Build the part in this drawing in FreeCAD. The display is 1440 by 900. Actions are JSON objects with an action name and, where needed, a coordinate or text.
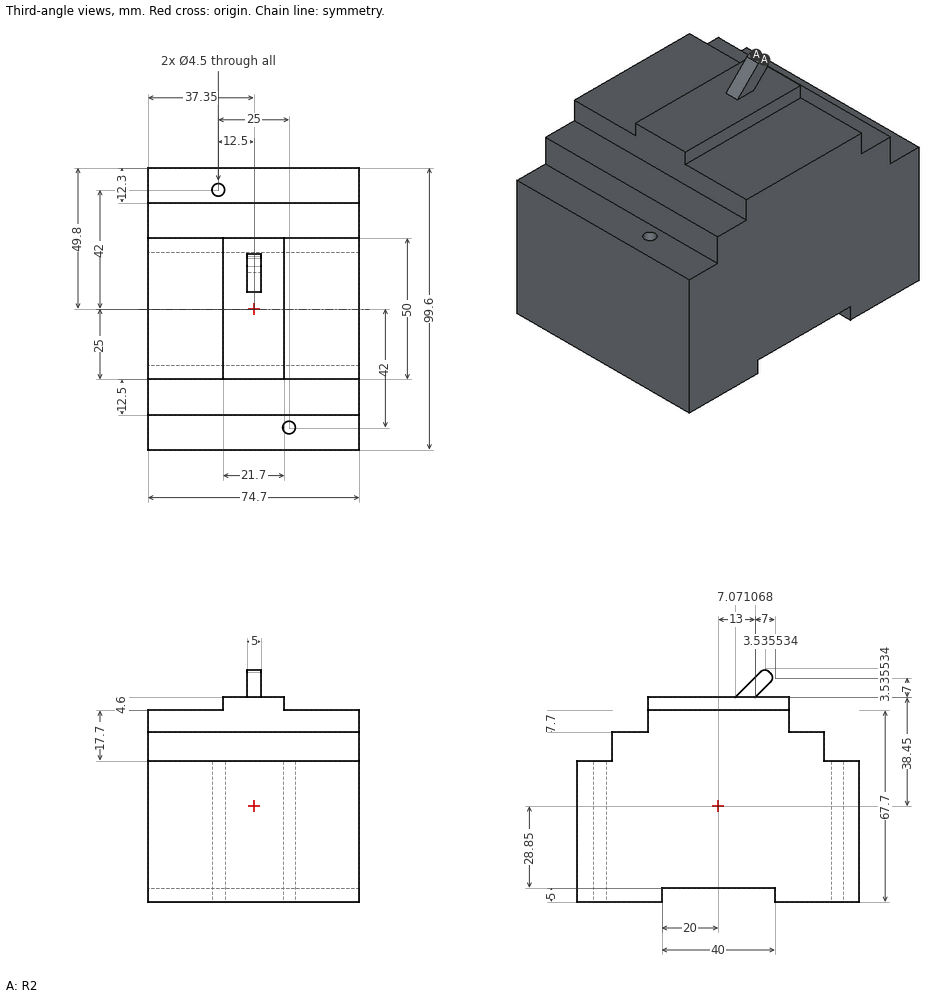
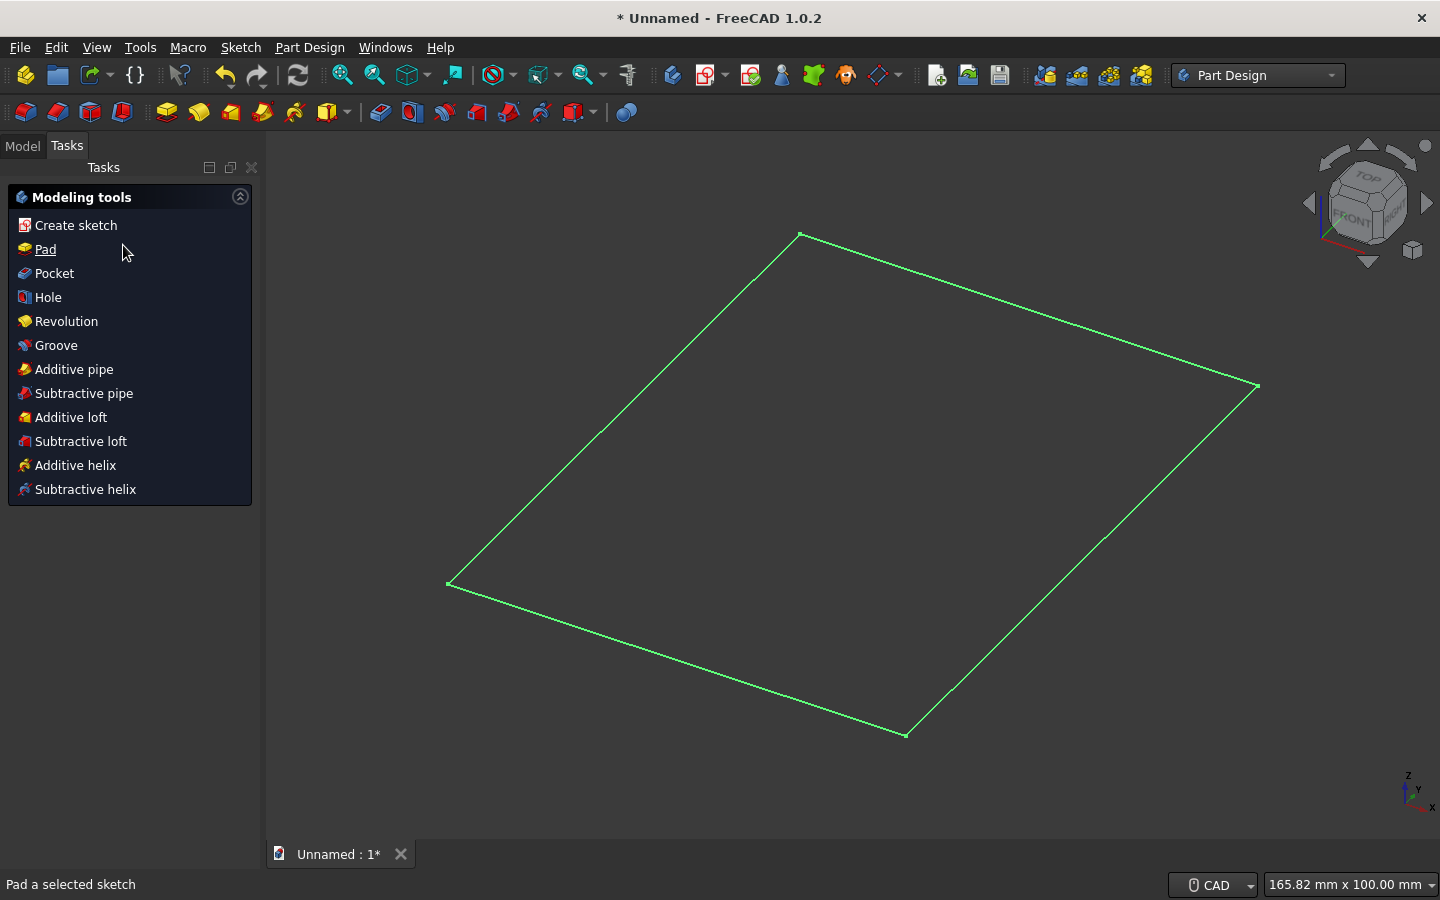
{"action": "left_click", "coordinate": [168, 112]}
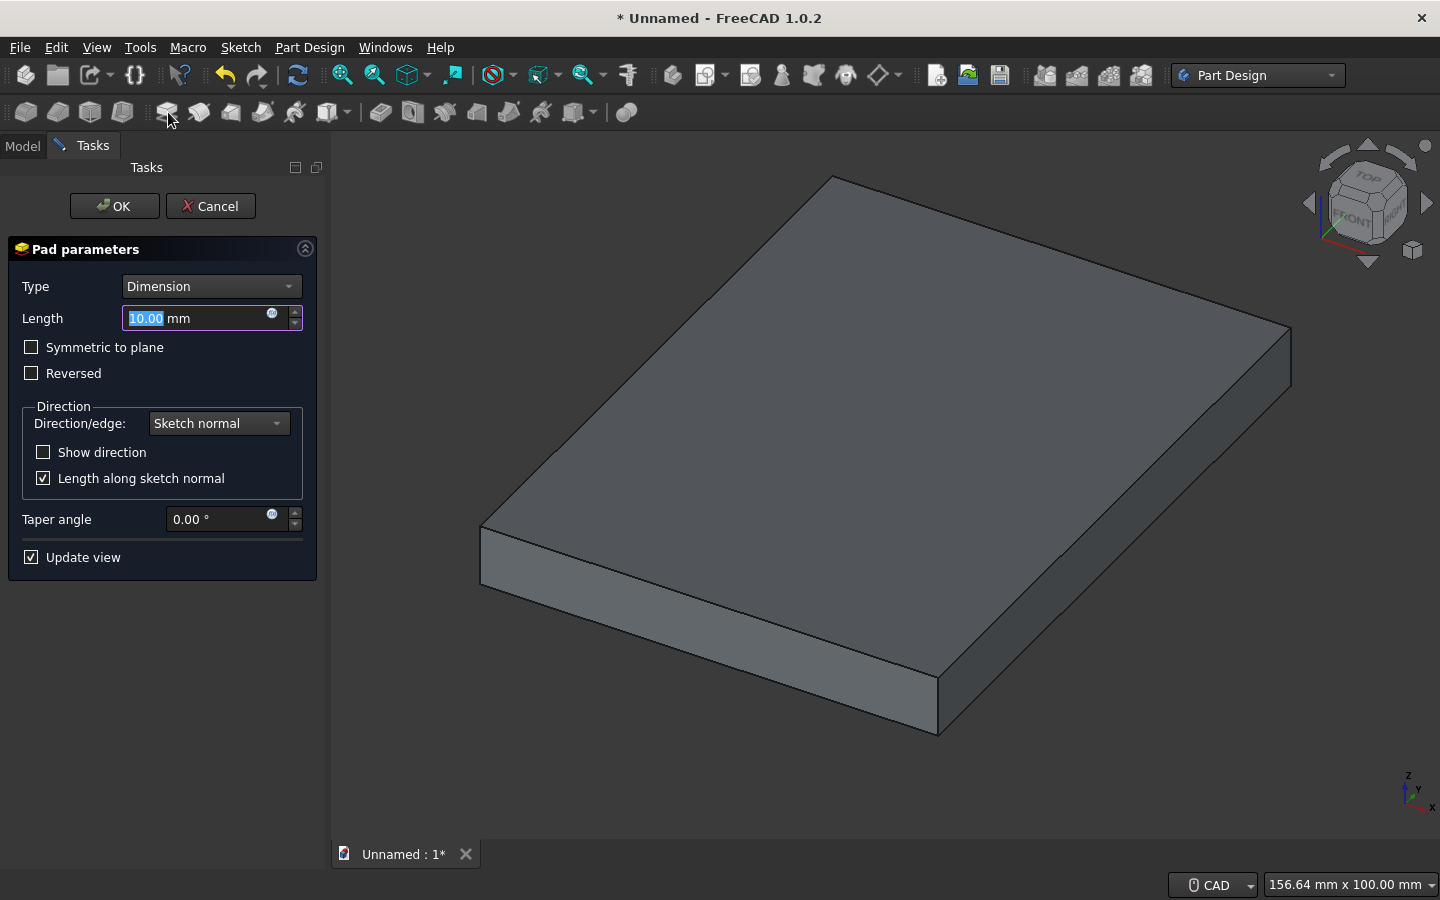
{"action": "type", "text": "67.7"}
{"action": "key", "text": "Tab"}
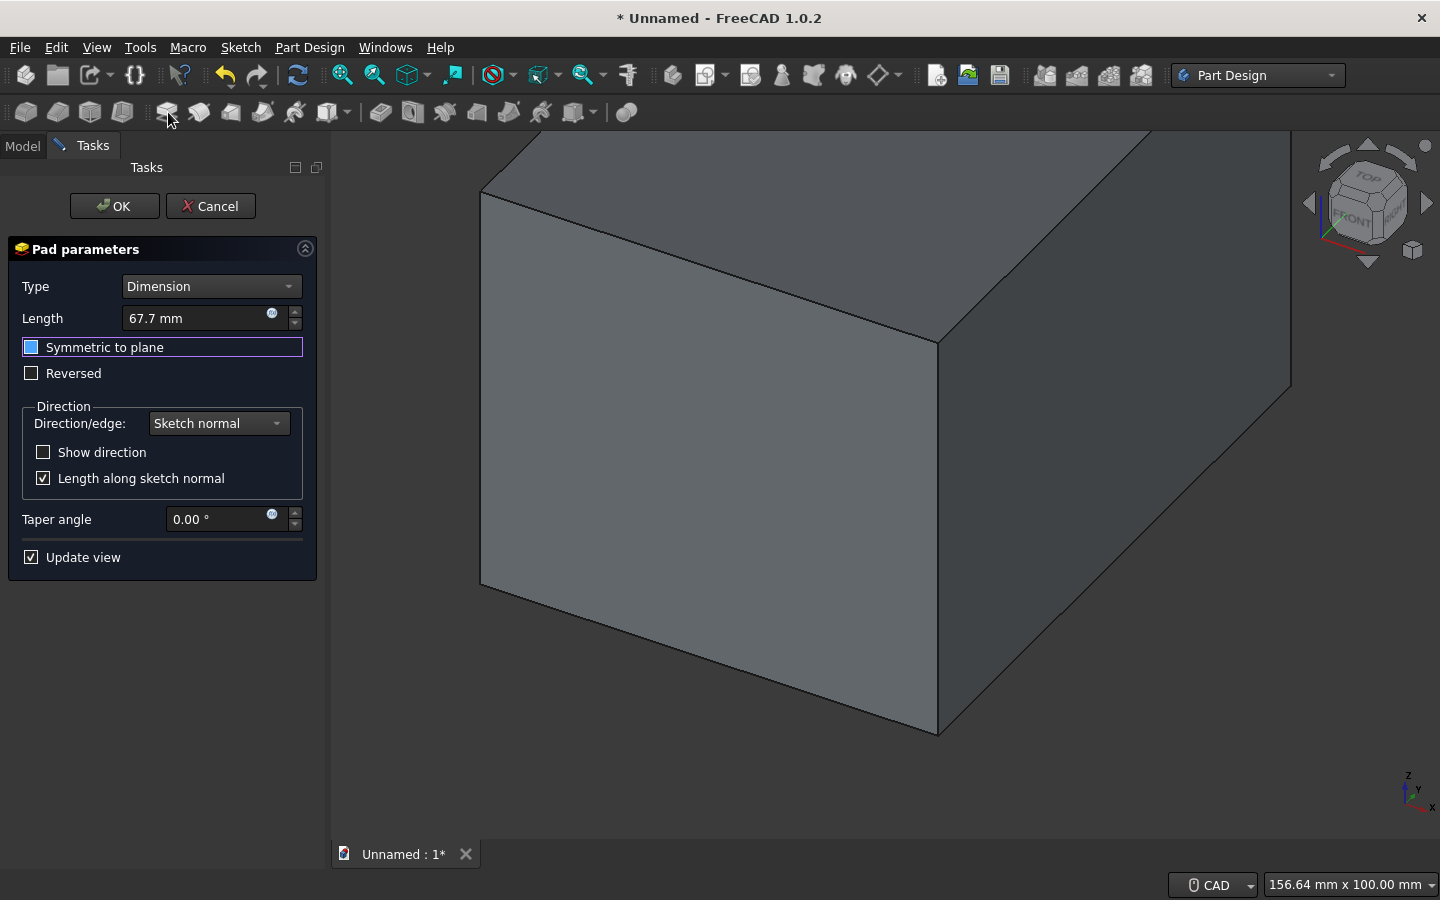
{"action": "left_click", "coordinate": [30, 347]}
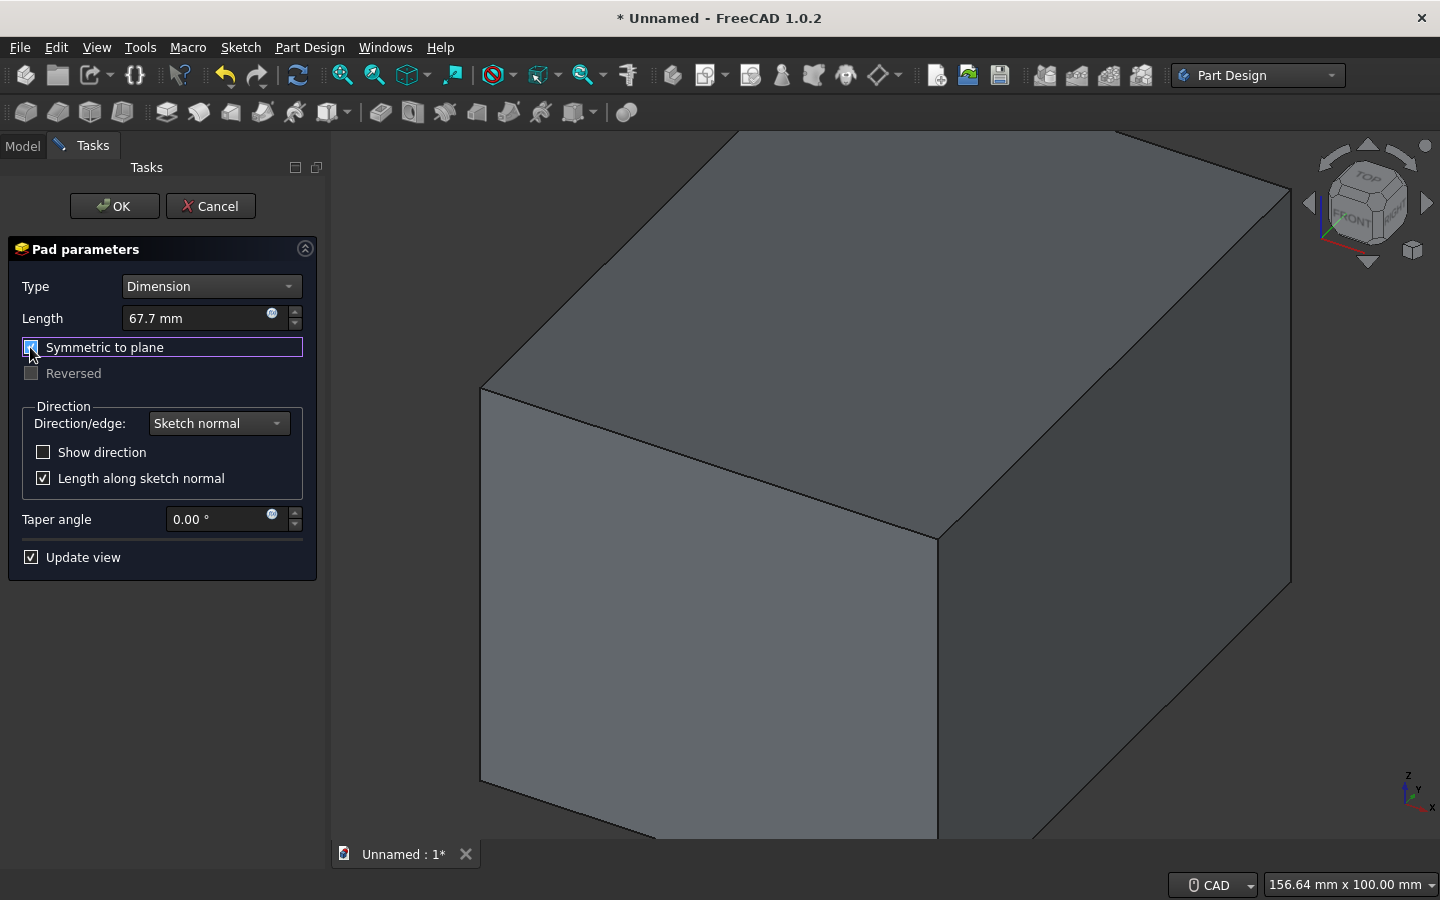
{"action": "left_click", "coordinate": [115, 206]}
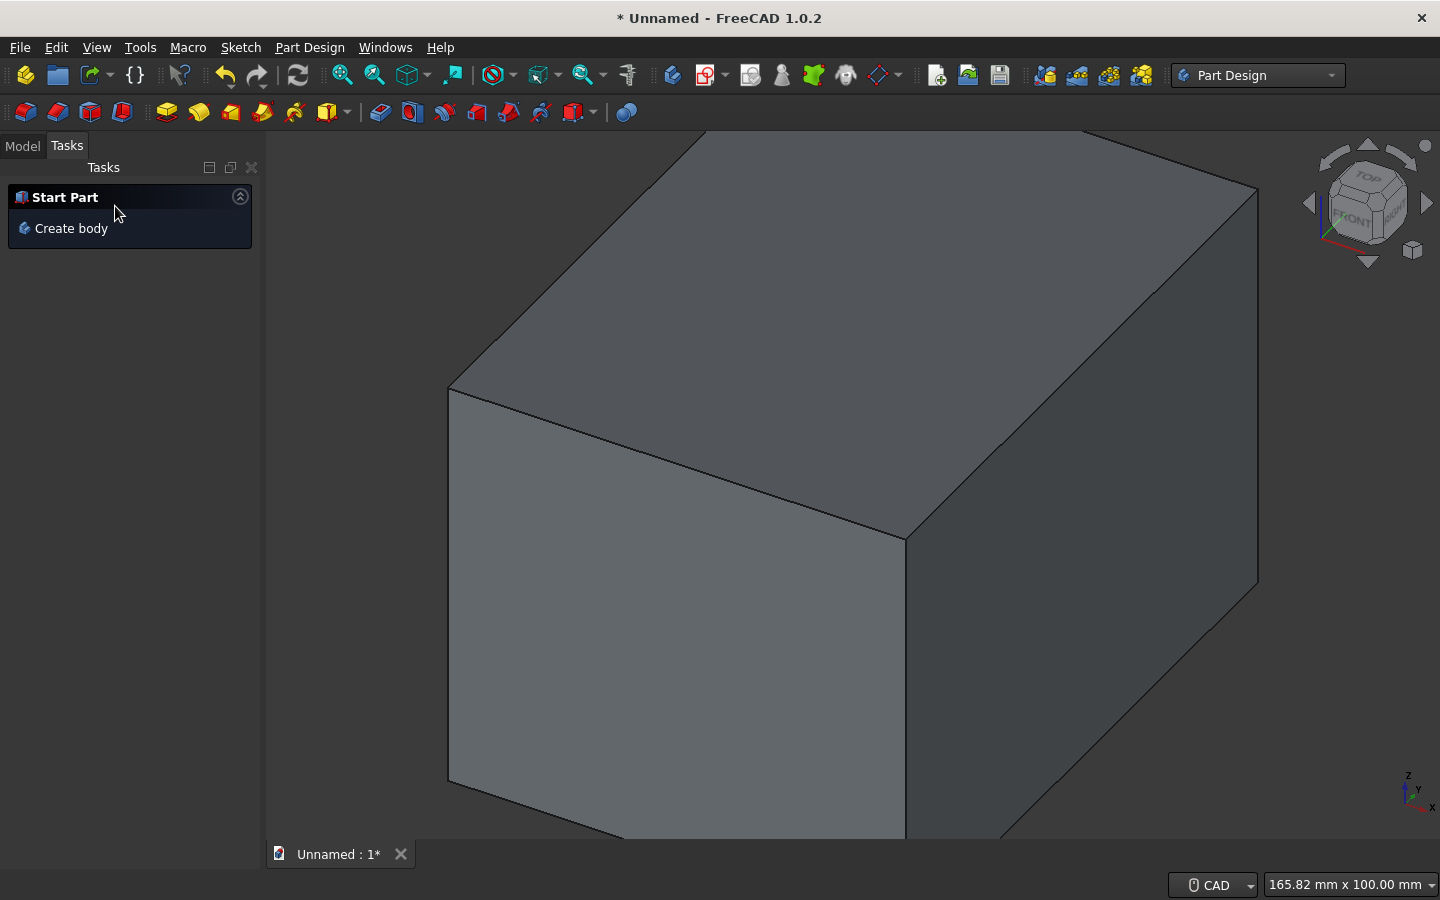
{"action": "left_click", "coordinate": [344, 76]}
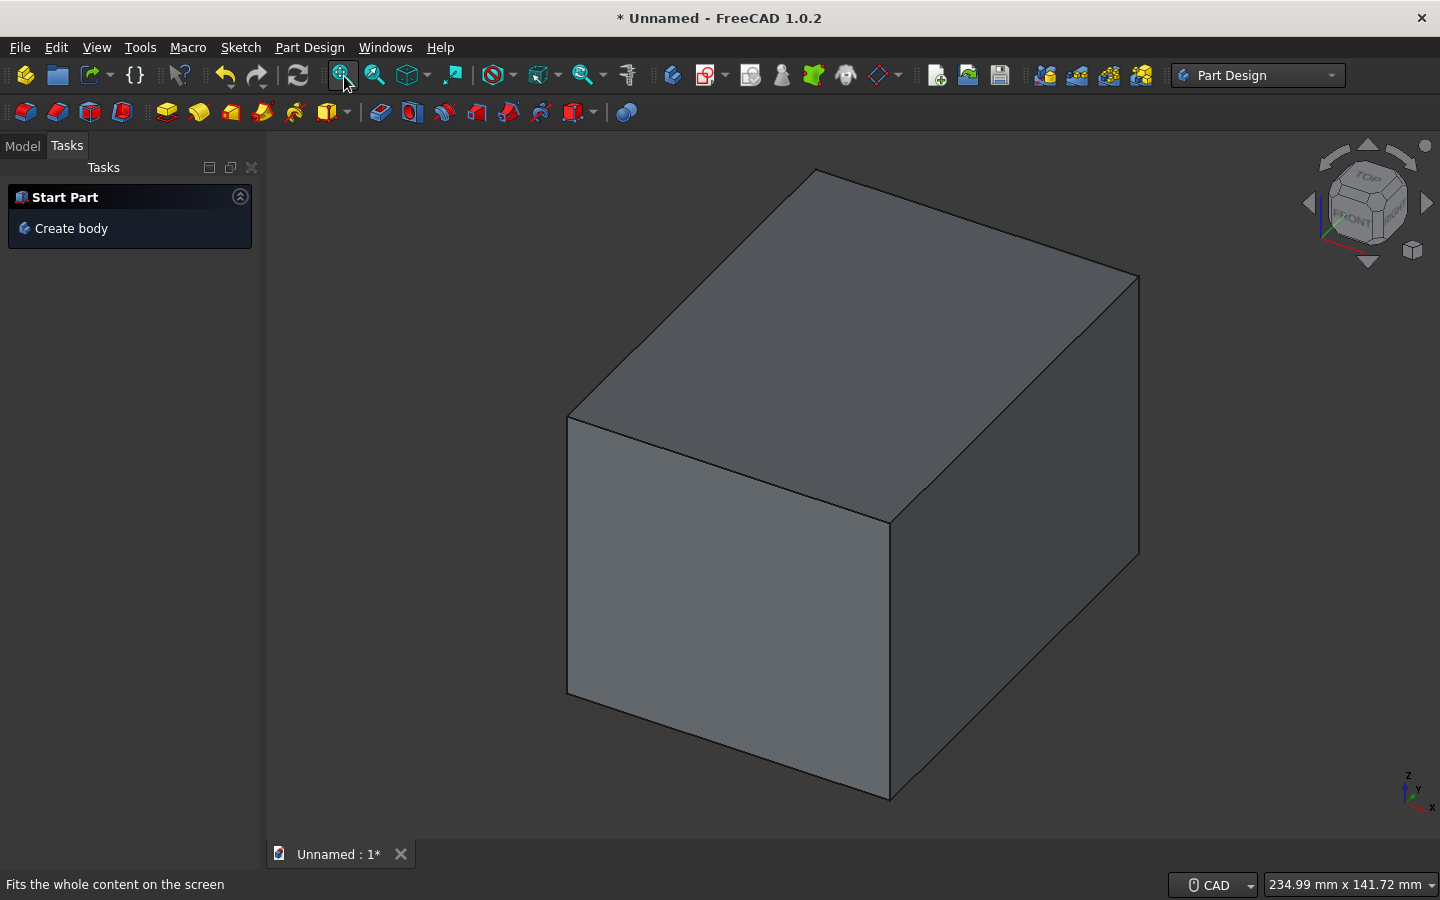
{"action": "left_click", "coordinate": [853, 345]}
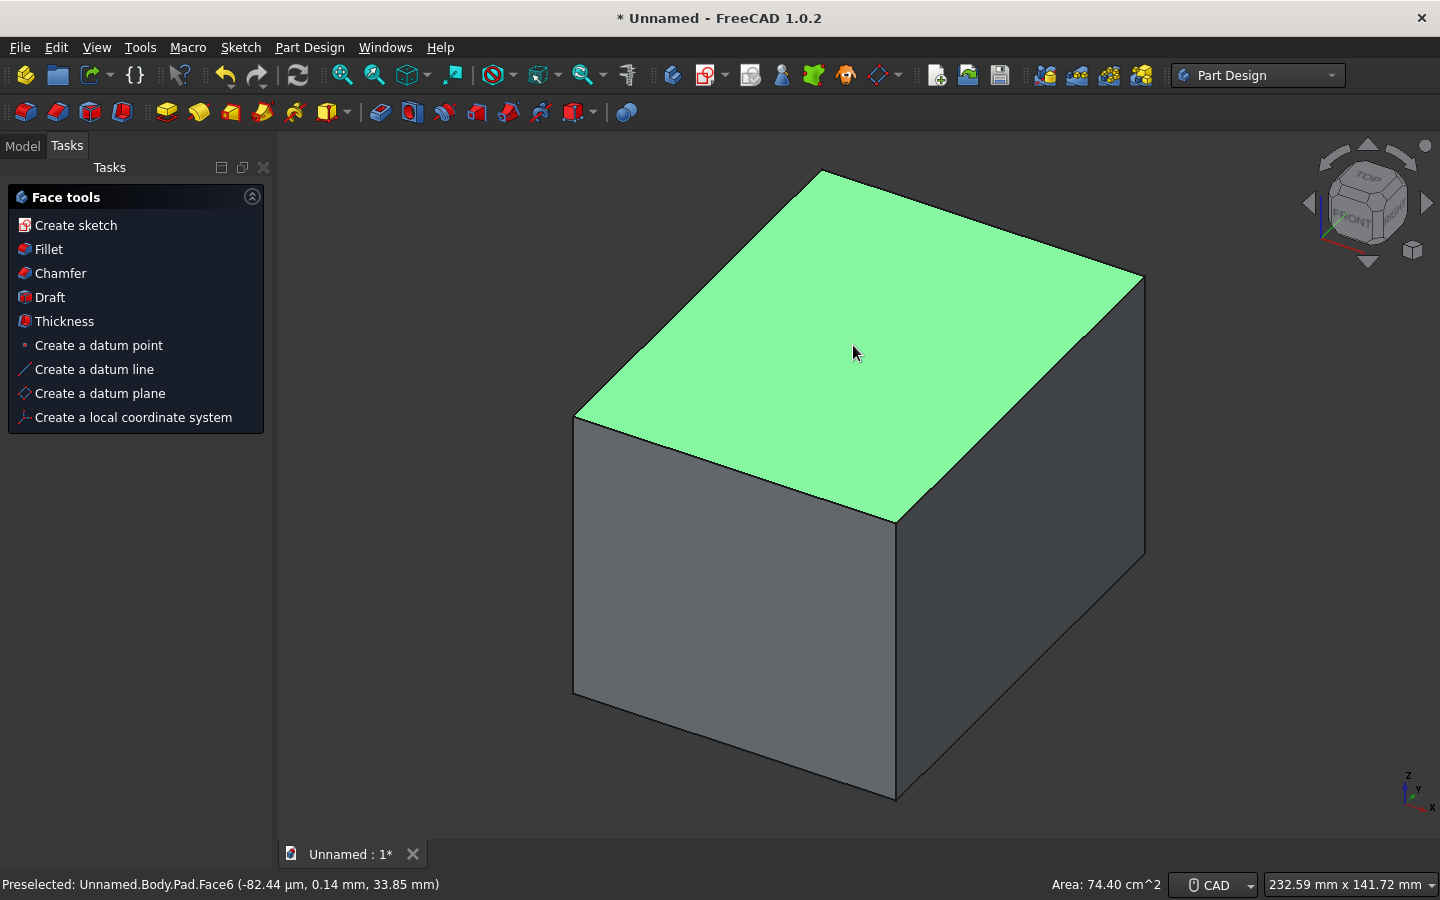
{"action": "left_click", "coordinate": [706, 76]}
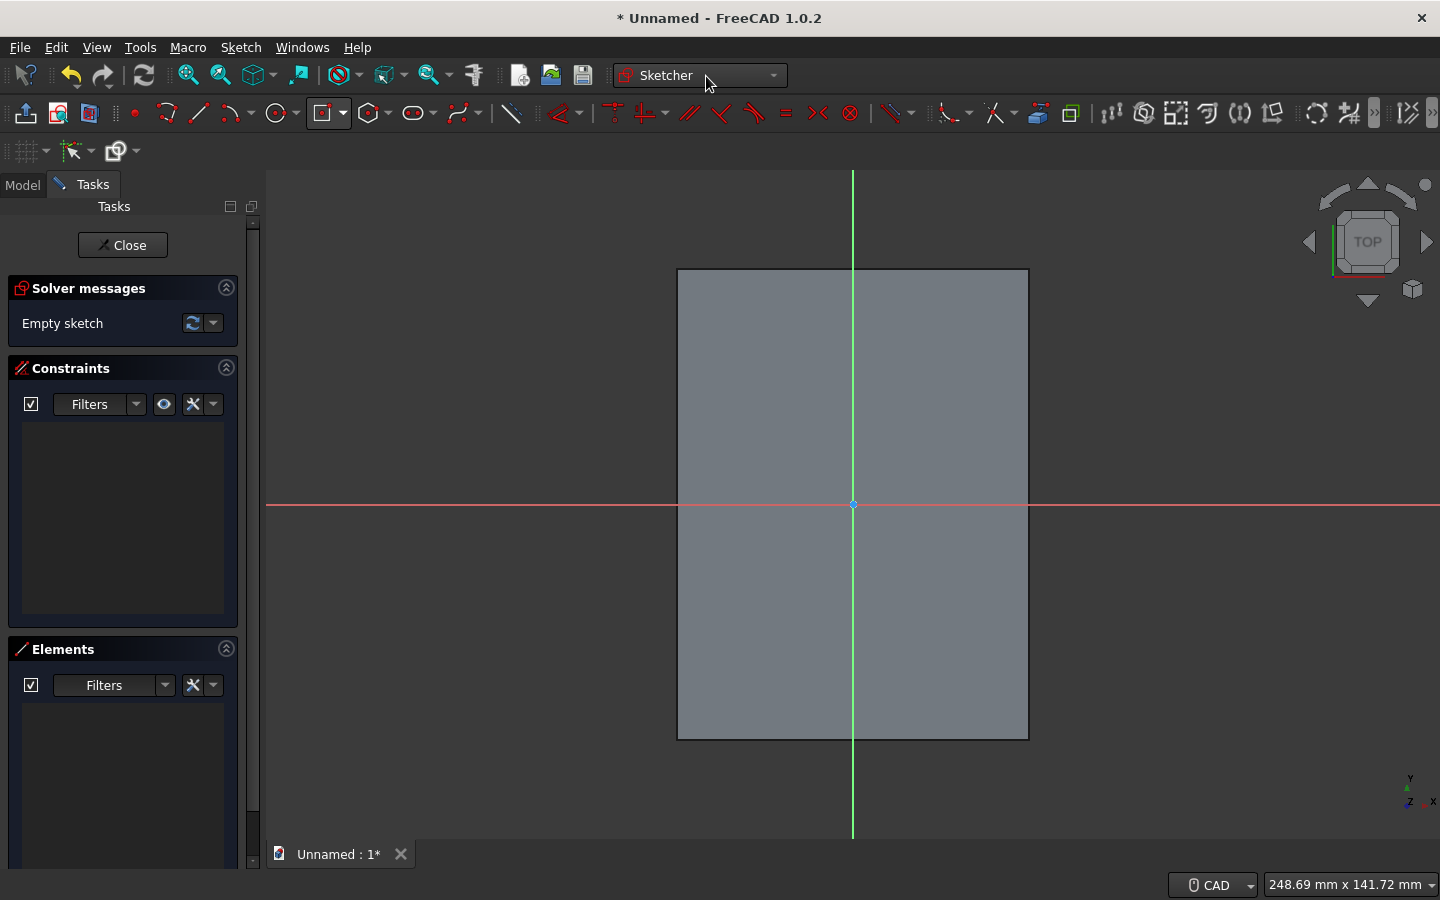
{"action": "key", "text": "g c"}